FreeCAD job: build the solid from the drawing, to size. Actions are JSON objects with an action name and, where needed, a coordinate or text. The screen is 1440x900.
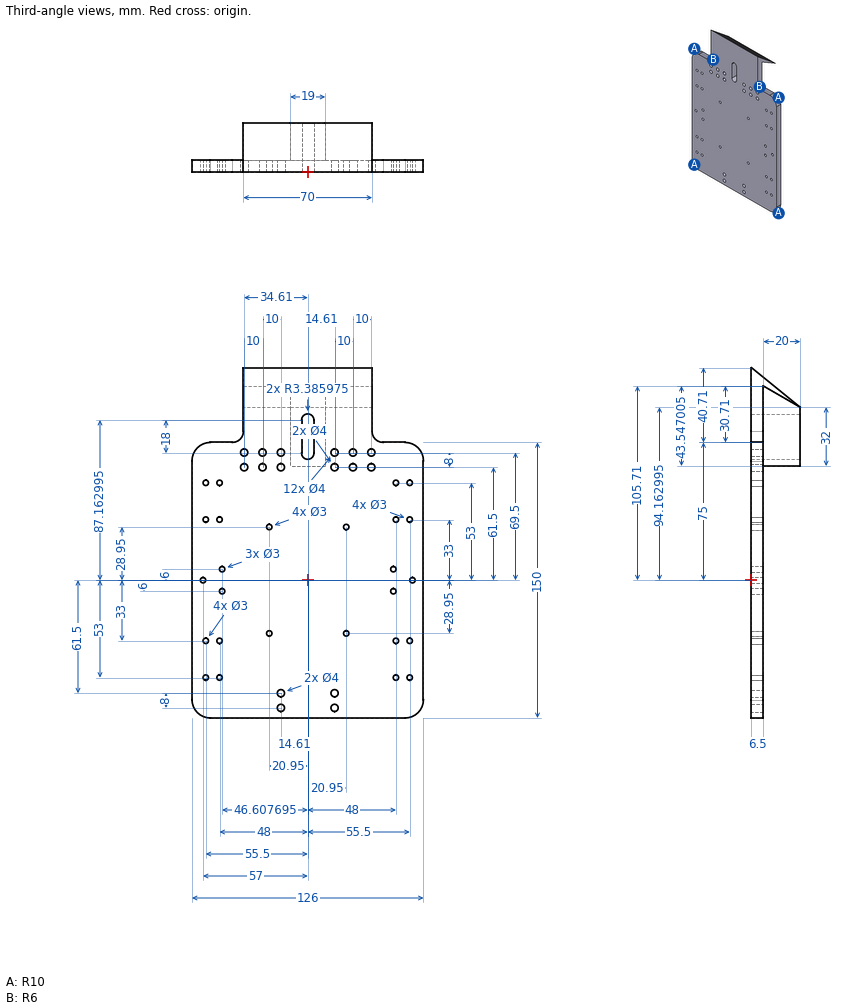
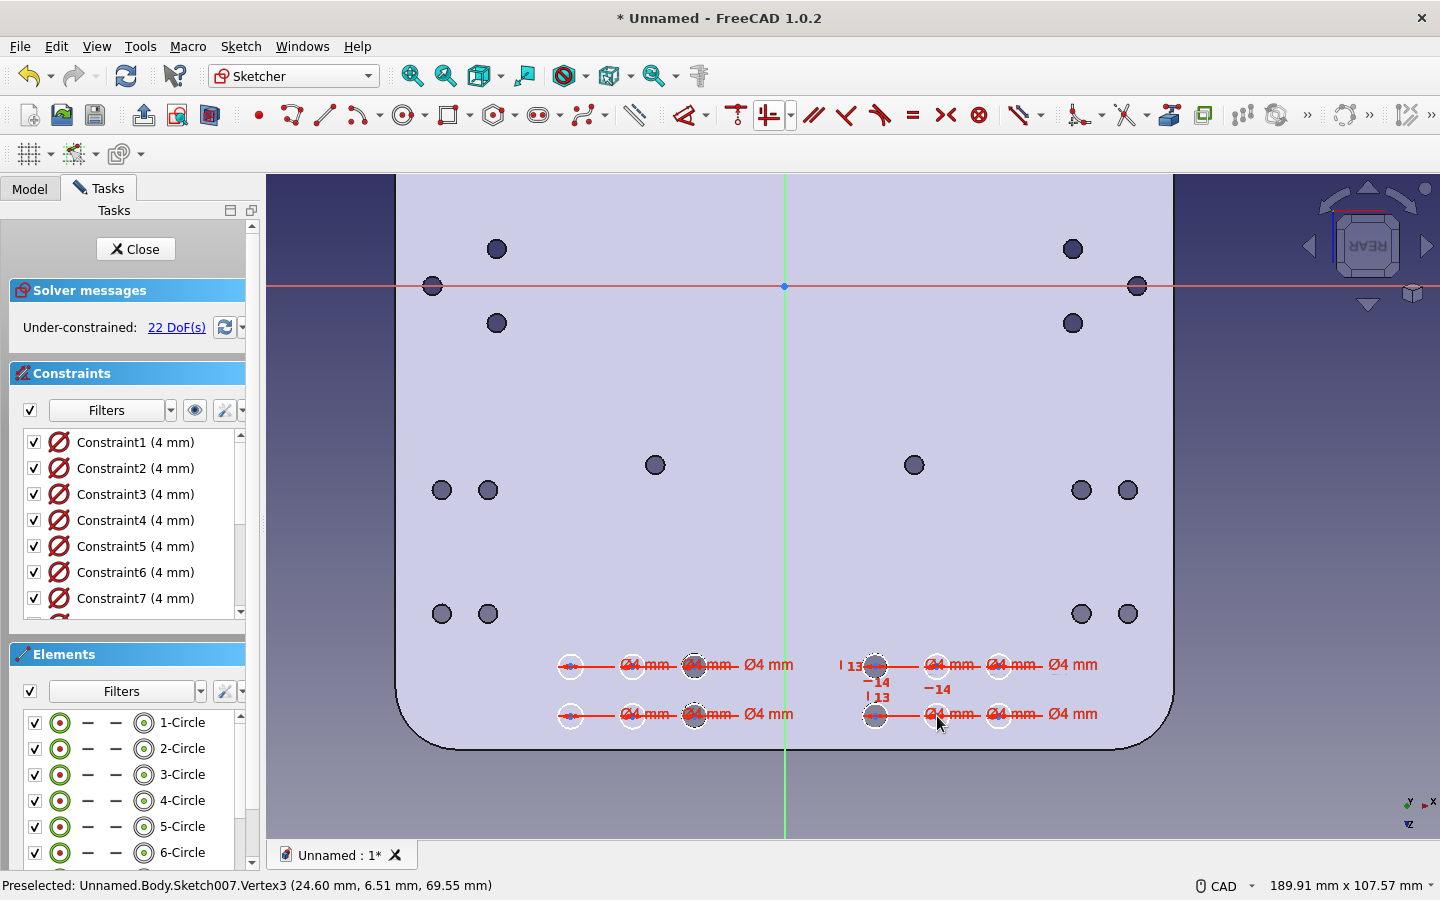
{"action": "left_click", "coordinate": [937, 716]}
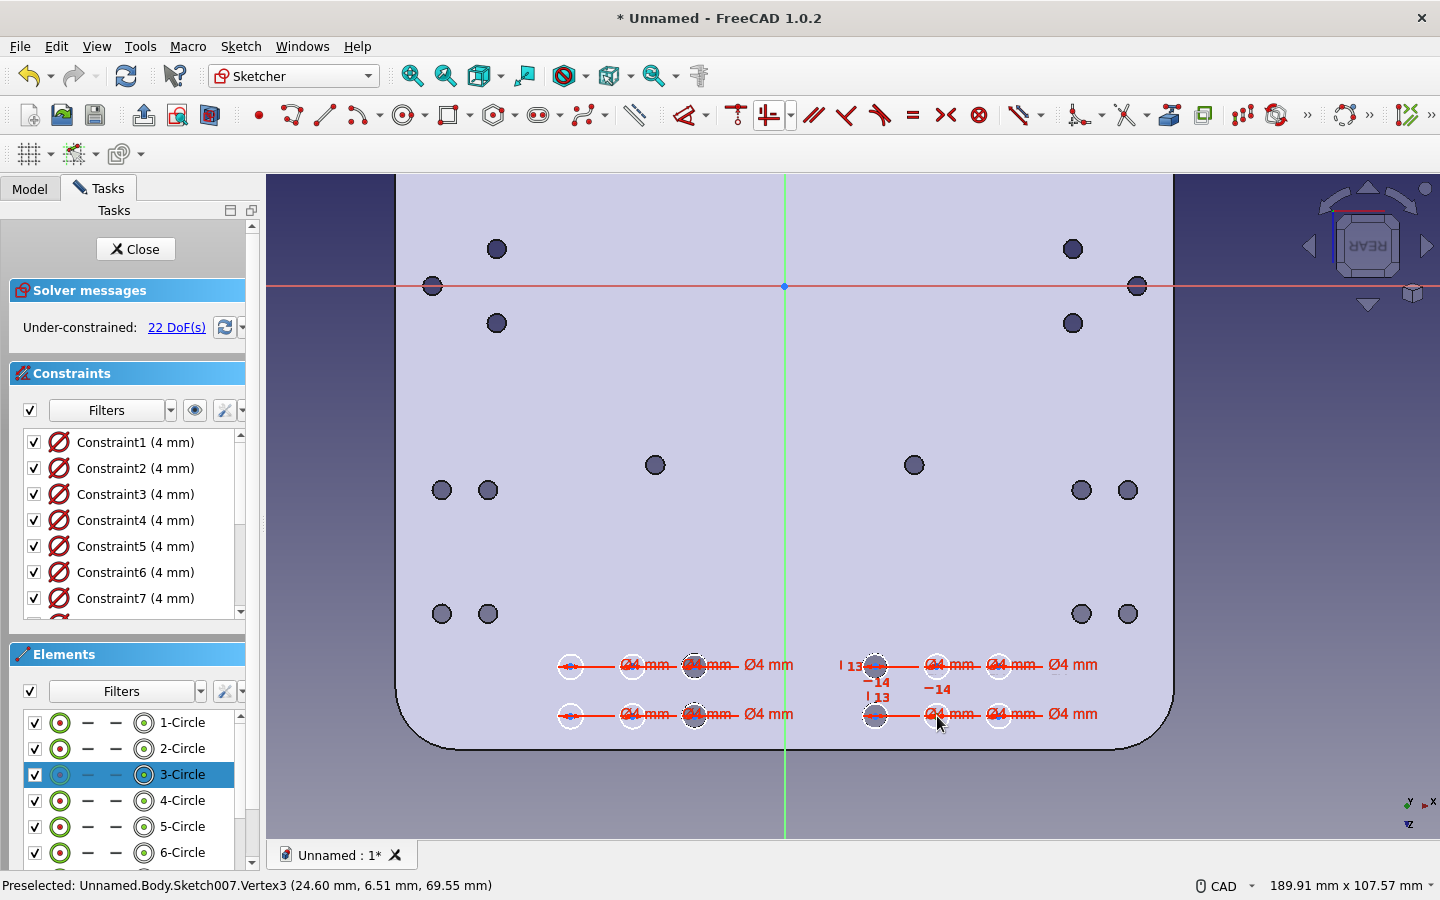
{"action": "left_click", "coordinate": [937, 667]}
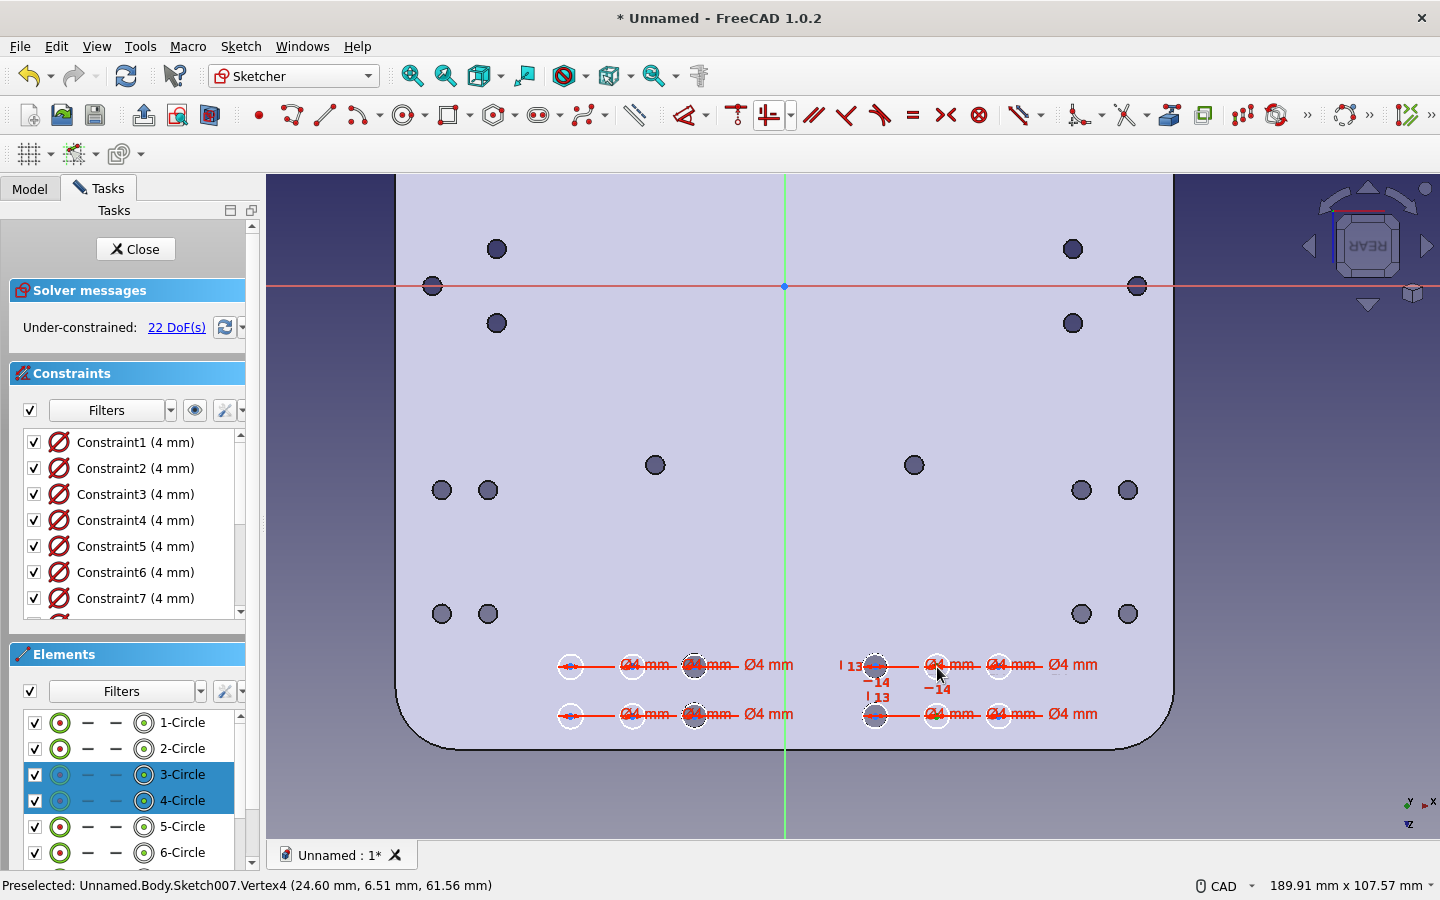
{"action": "key", "text": "v"}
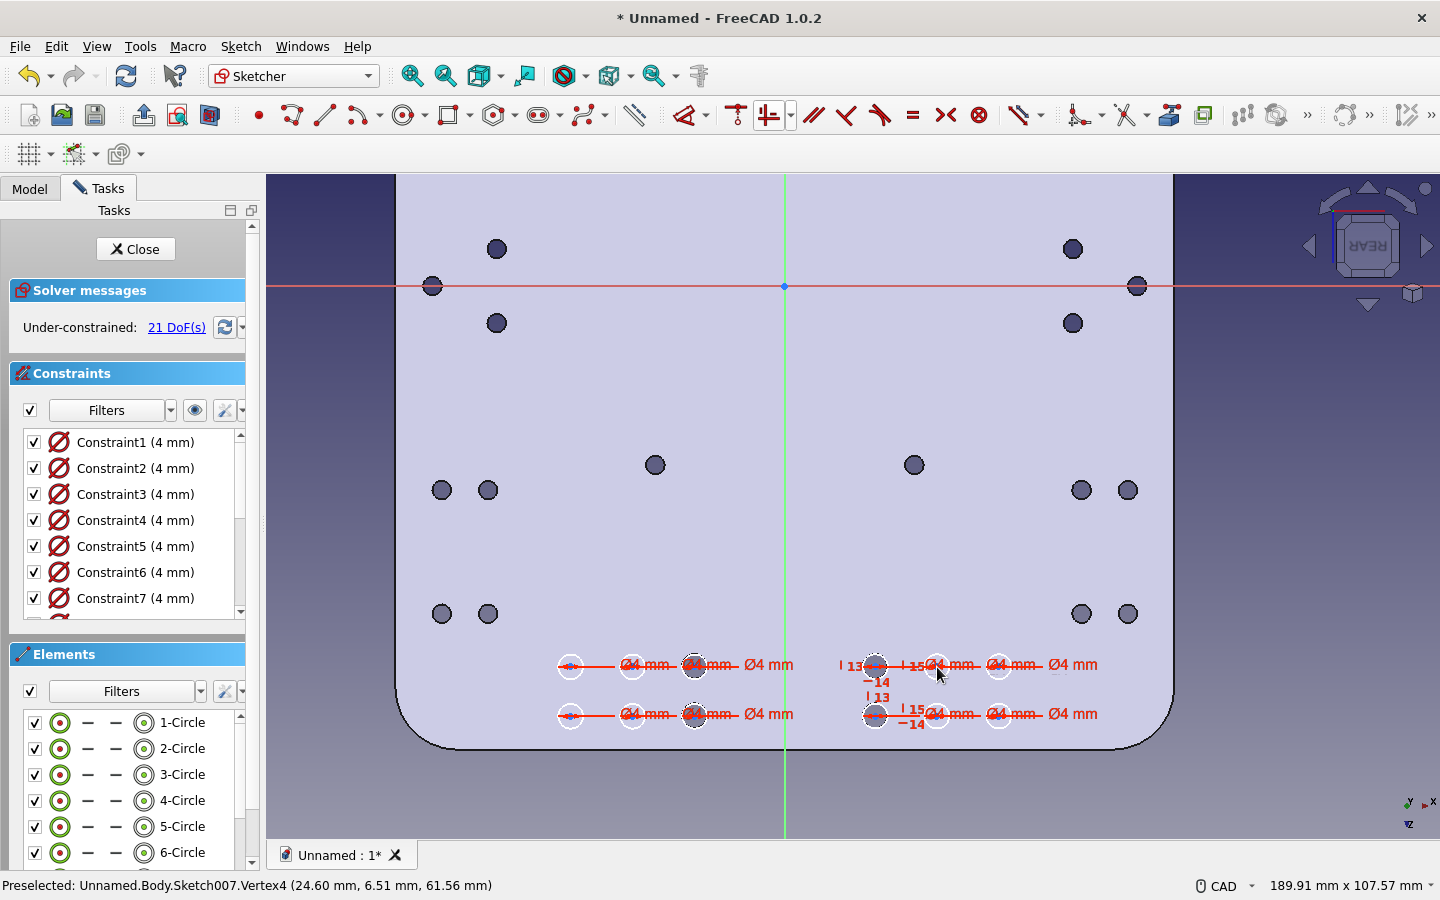
{"action": "left_click", "coordinate": [875, 667]}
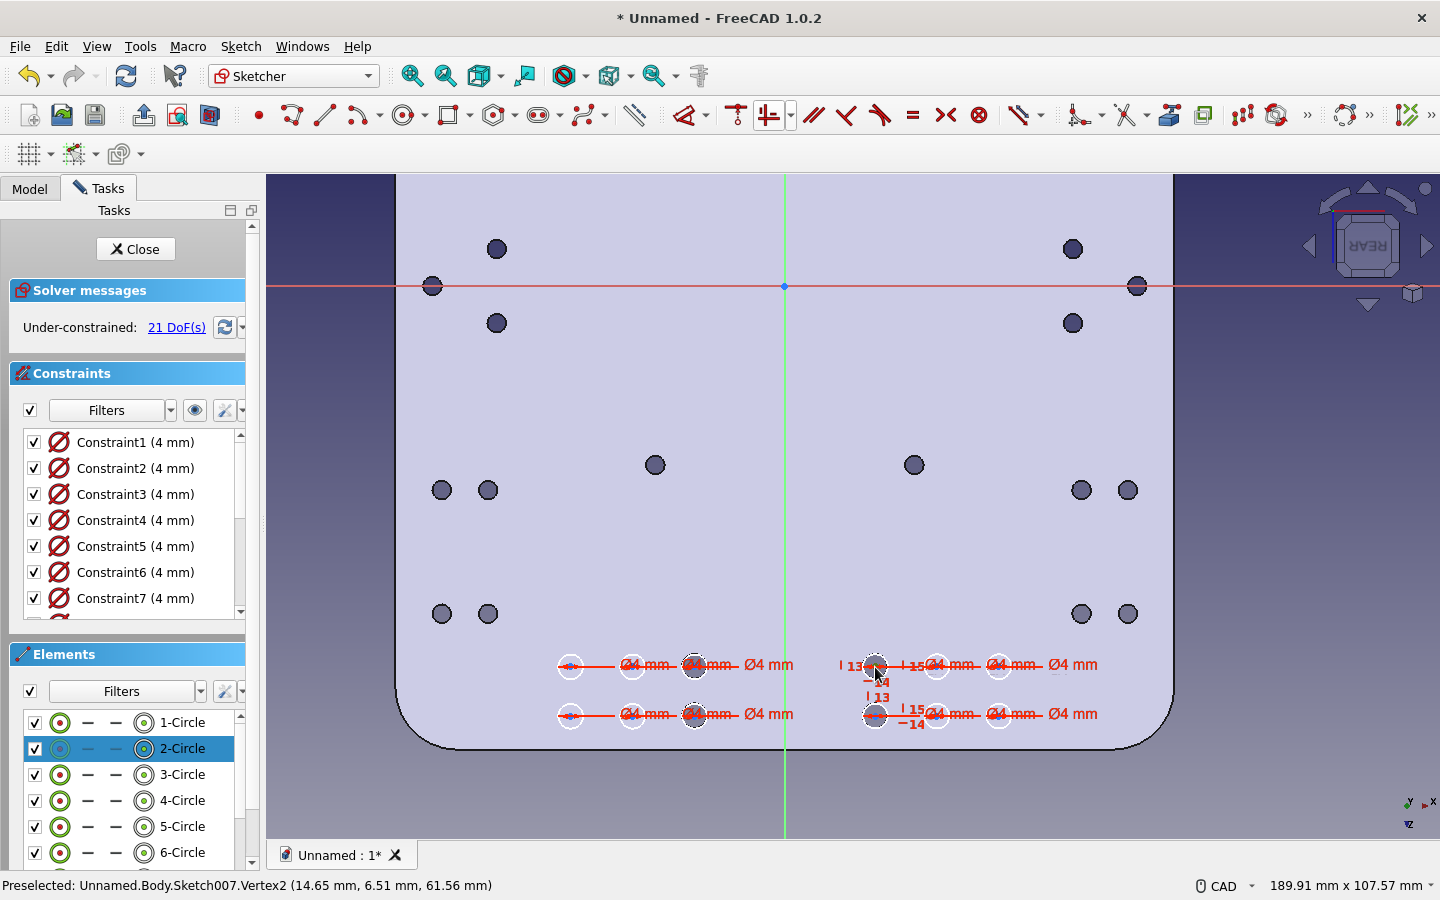
{"action": "left_click", "coordinate": [937, 667]}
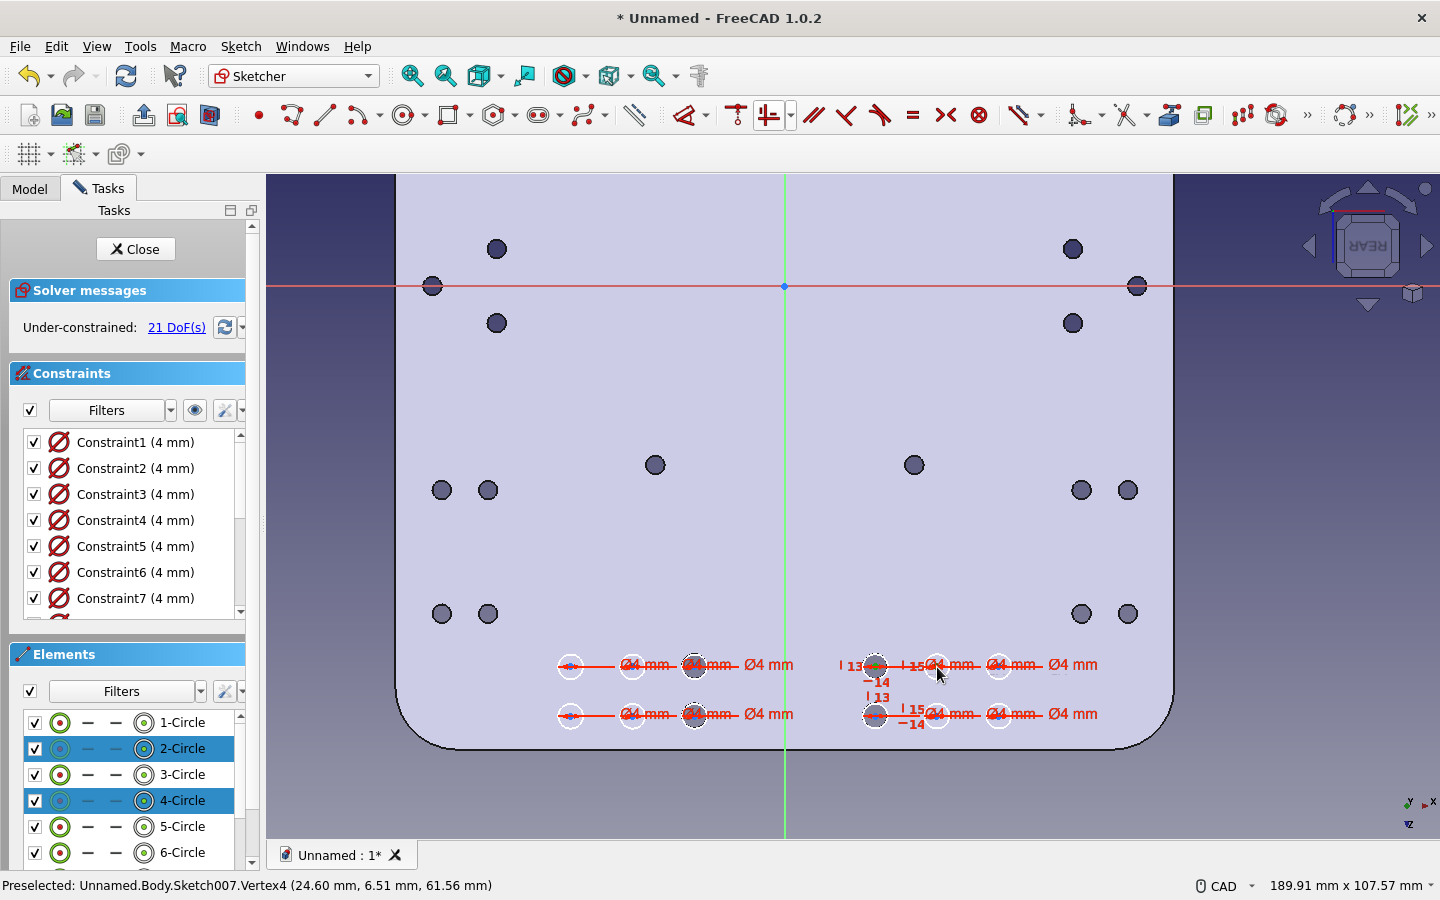
{"action": "key", "text": "h"}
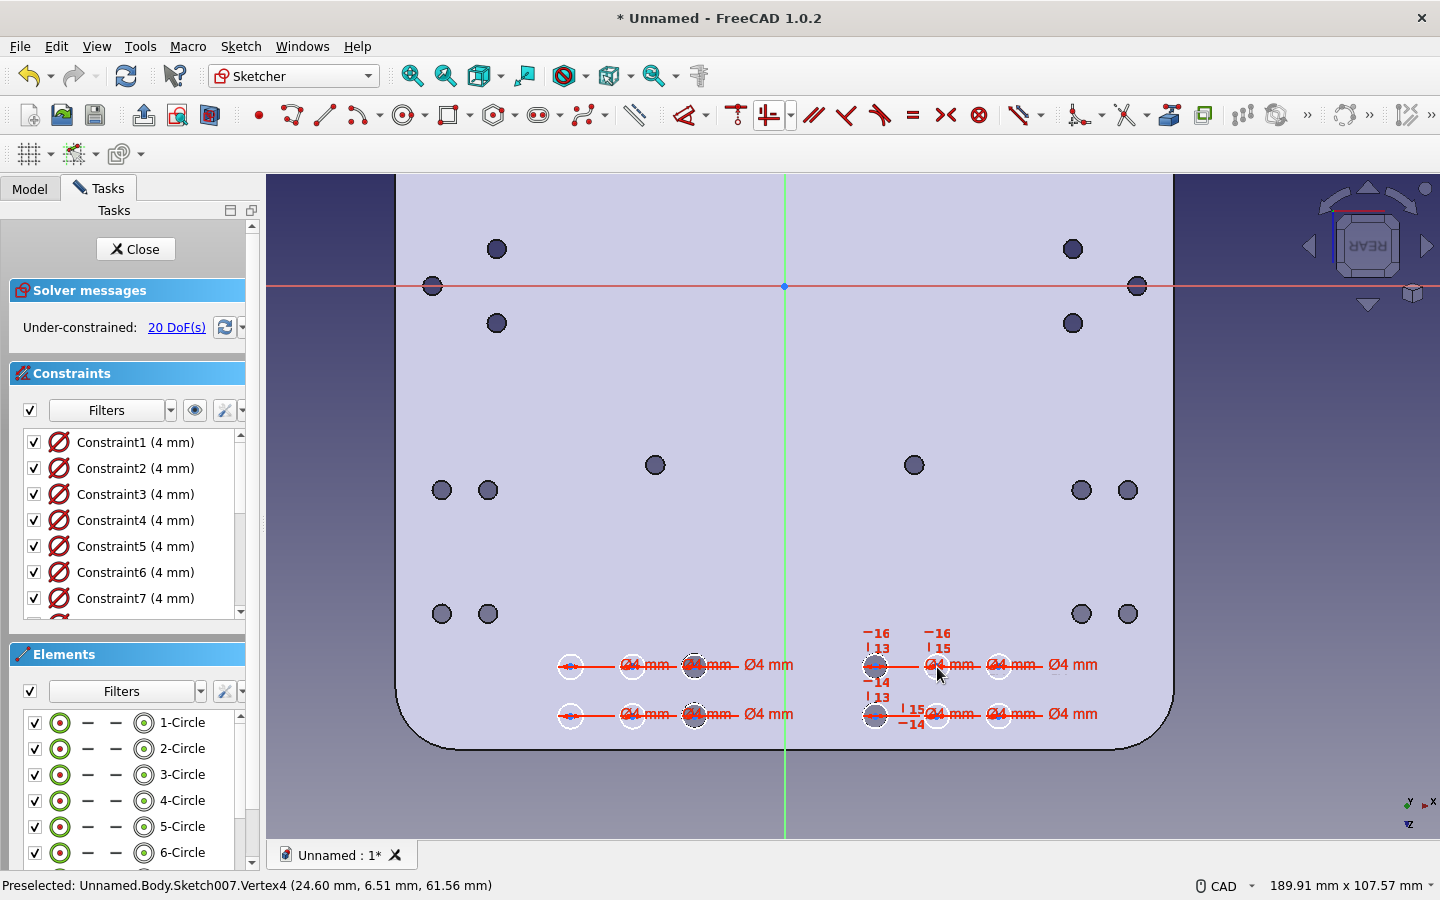
{"action": "left_click", "coordinate": [937, 716]}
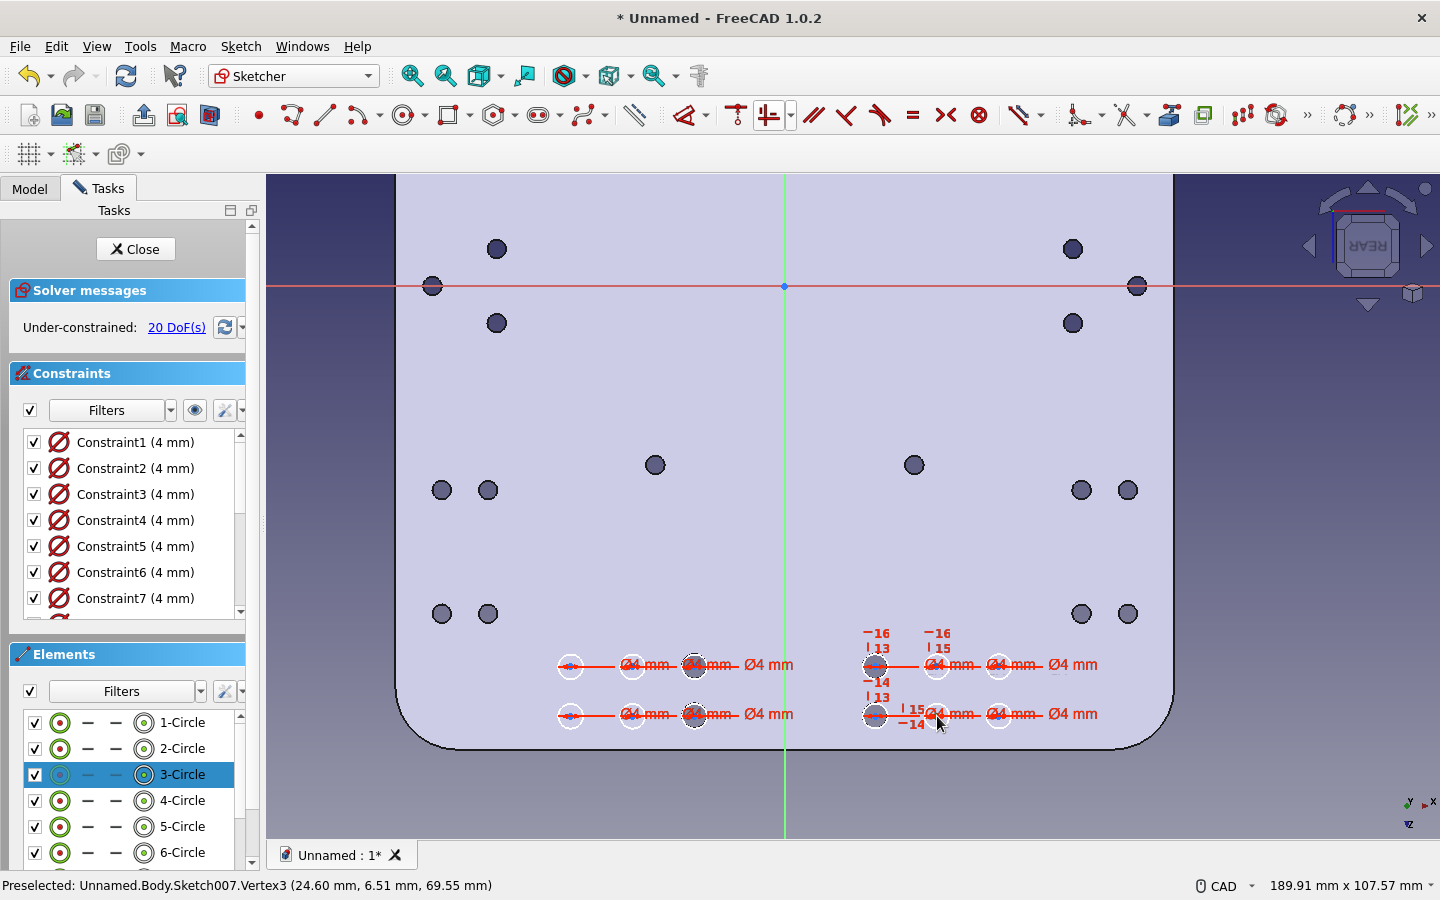
{"action": "left_click", "coordinate": [999, 716]}